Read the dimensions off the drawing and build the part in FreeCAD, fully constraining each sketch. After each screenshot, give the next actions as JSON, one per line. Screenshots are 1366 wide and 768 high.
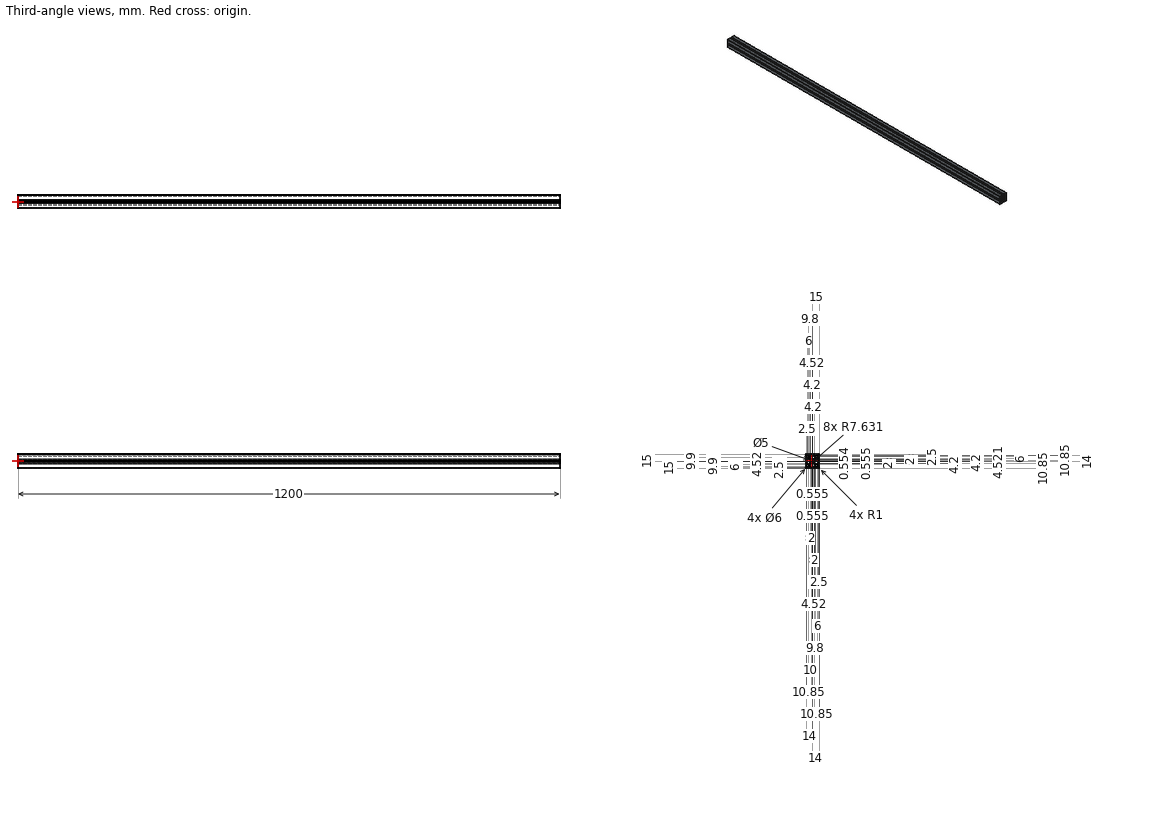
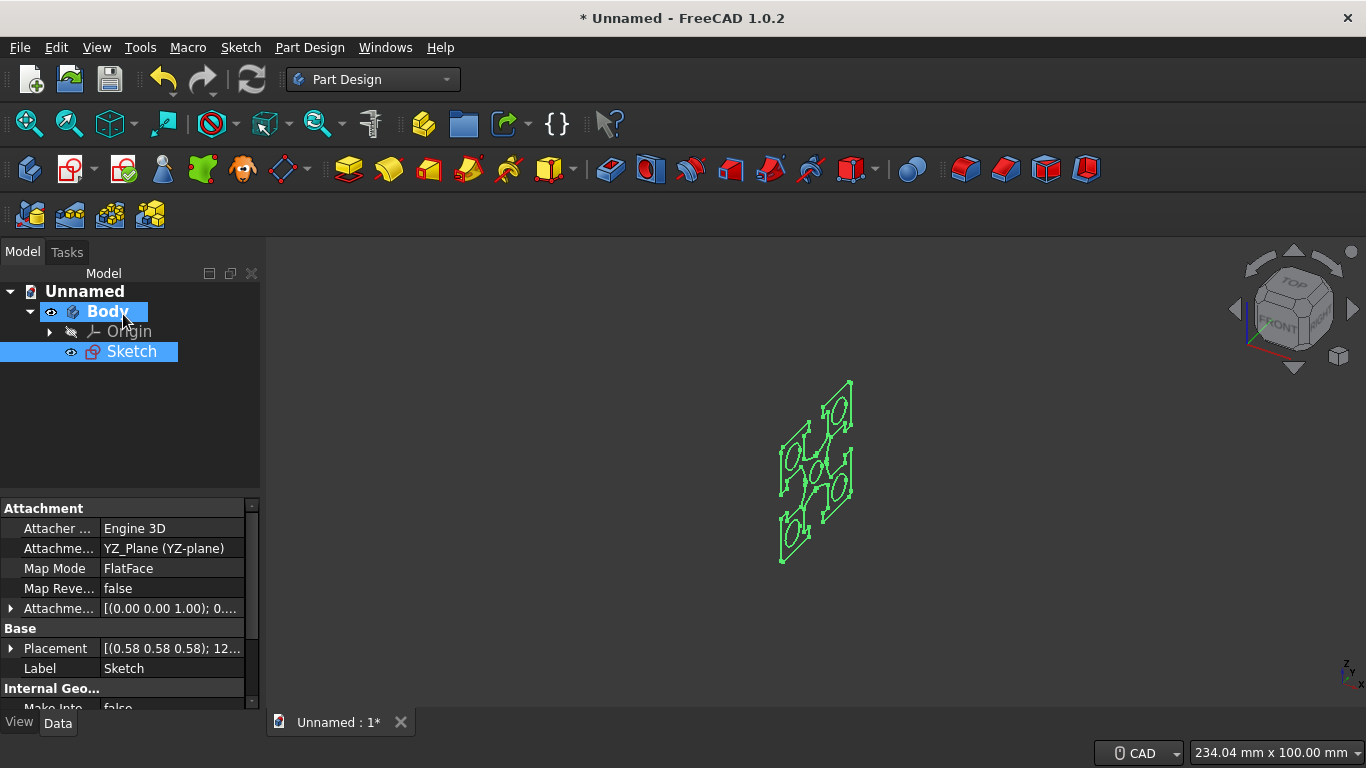
{"action": "left_click", "coordinate": [350, 170]}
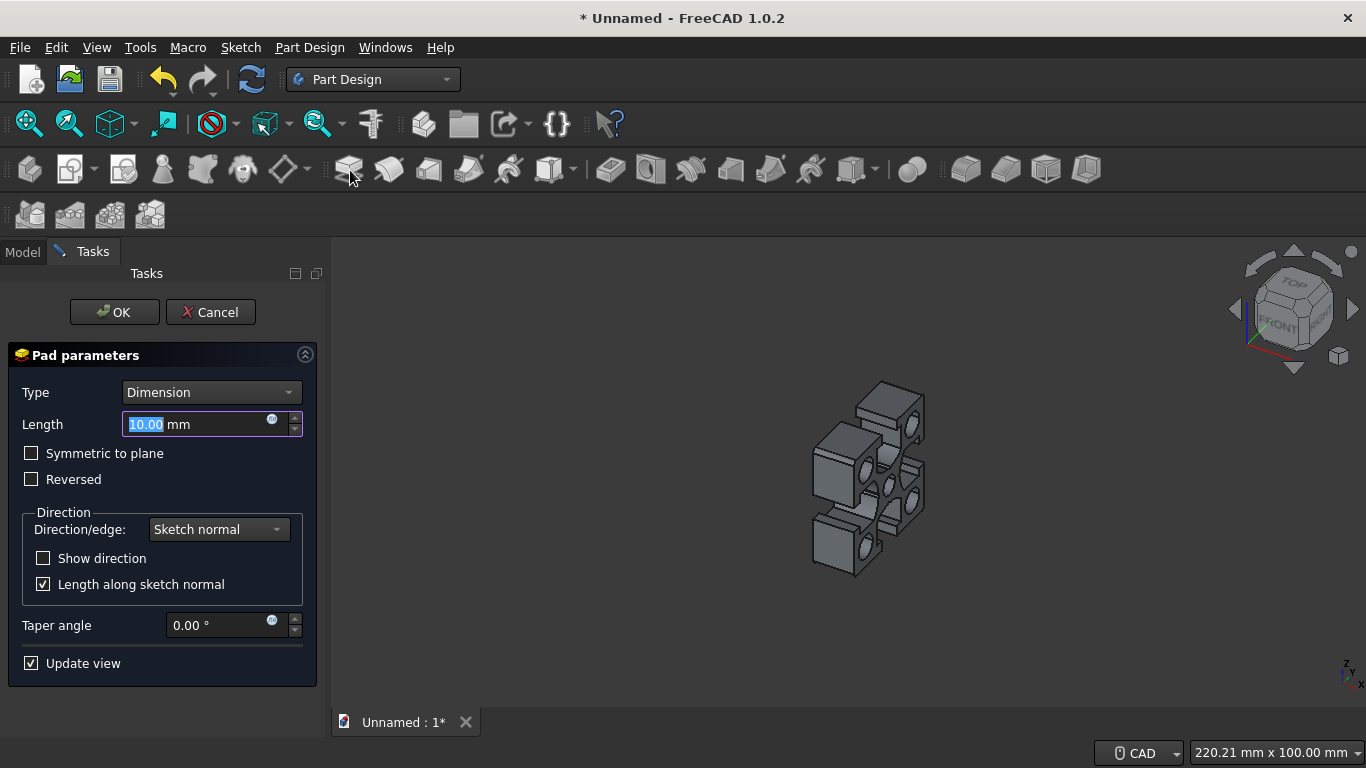
{"action": "type", "text": "1200"}
{"action": "key", "text": "Tab"}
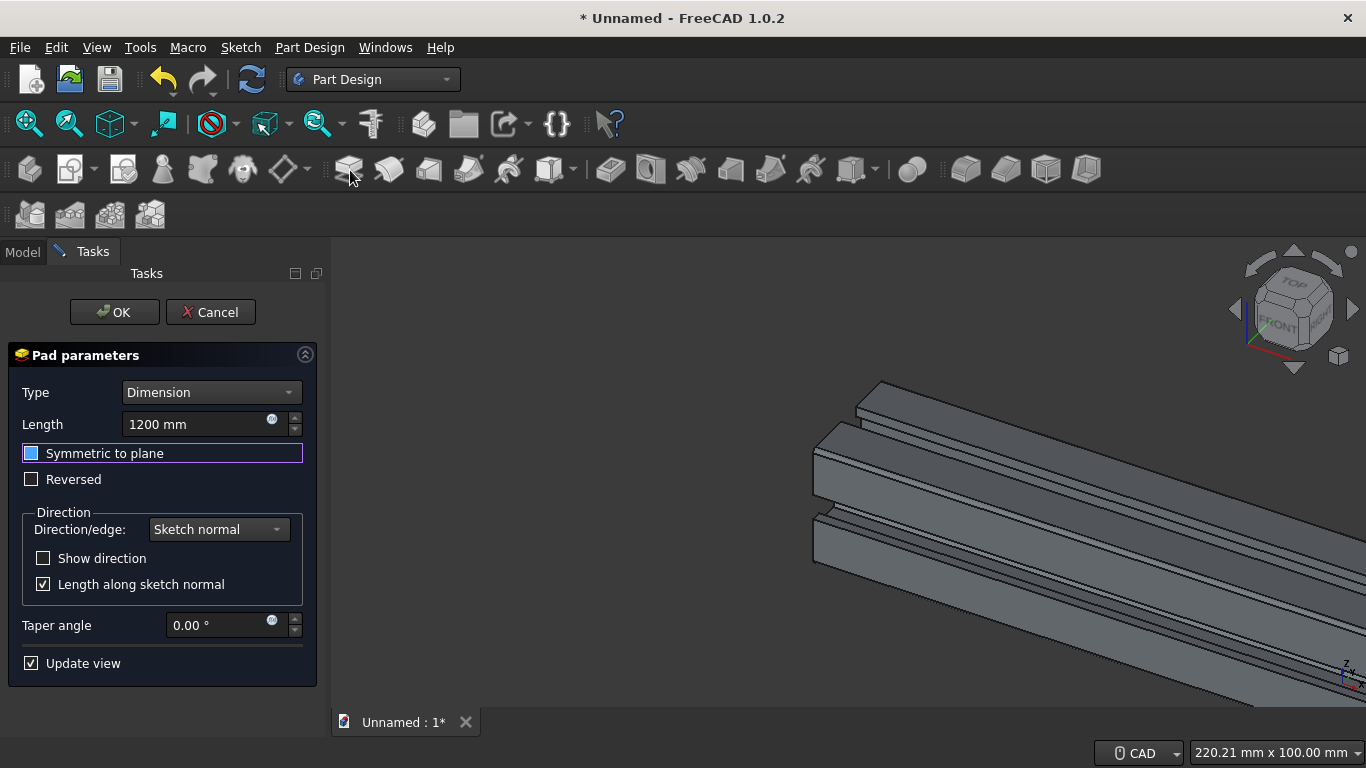
{"action": "left_click", "coordinate": [115, 312]}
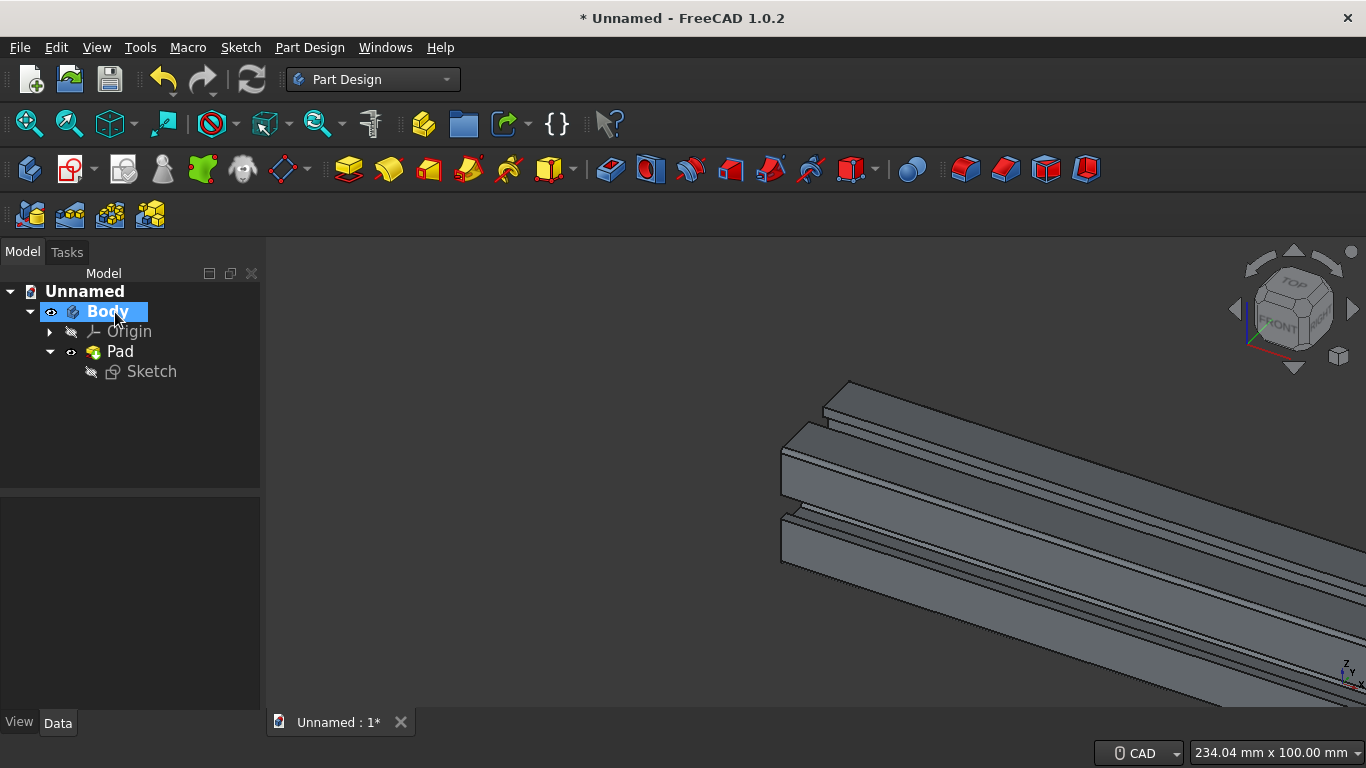
{"action": "key", "text": "0"}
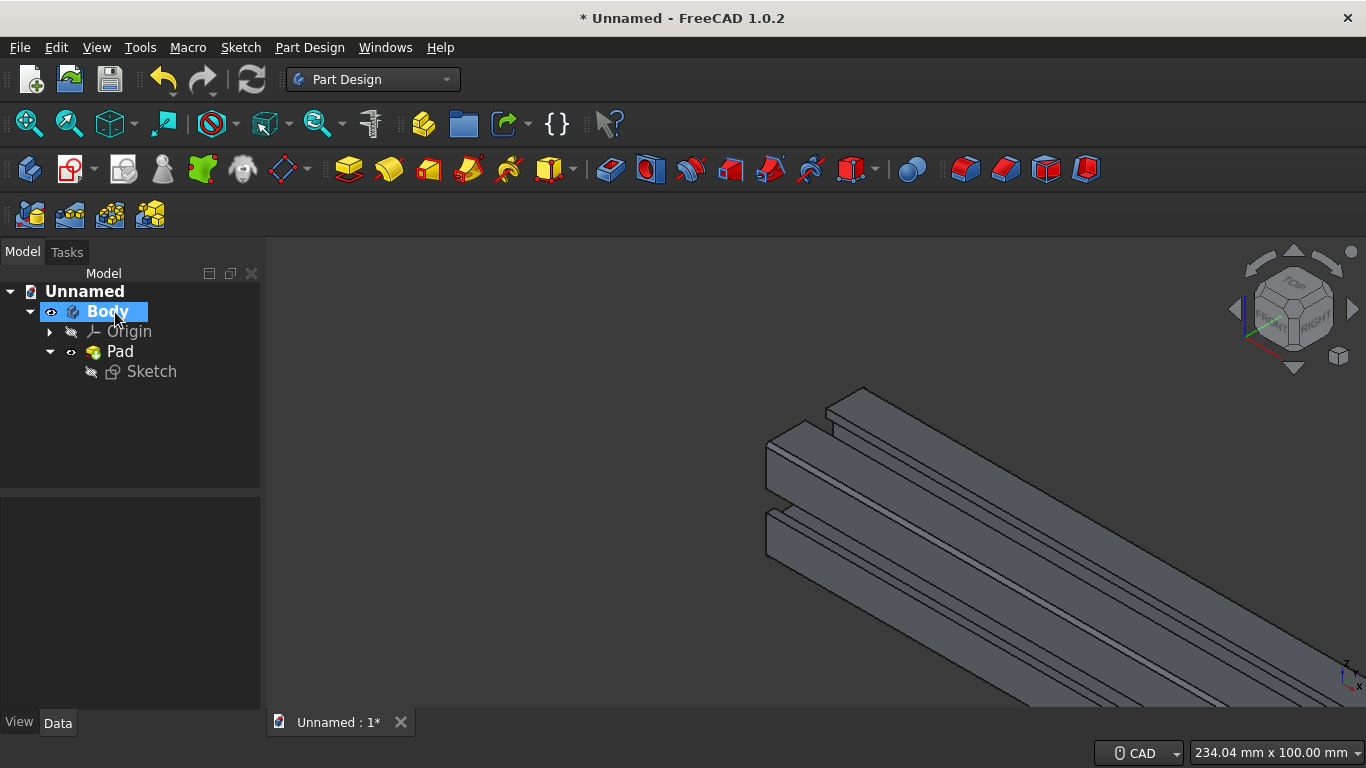
{"action": "left_click", "coordinate": [30, 124]}